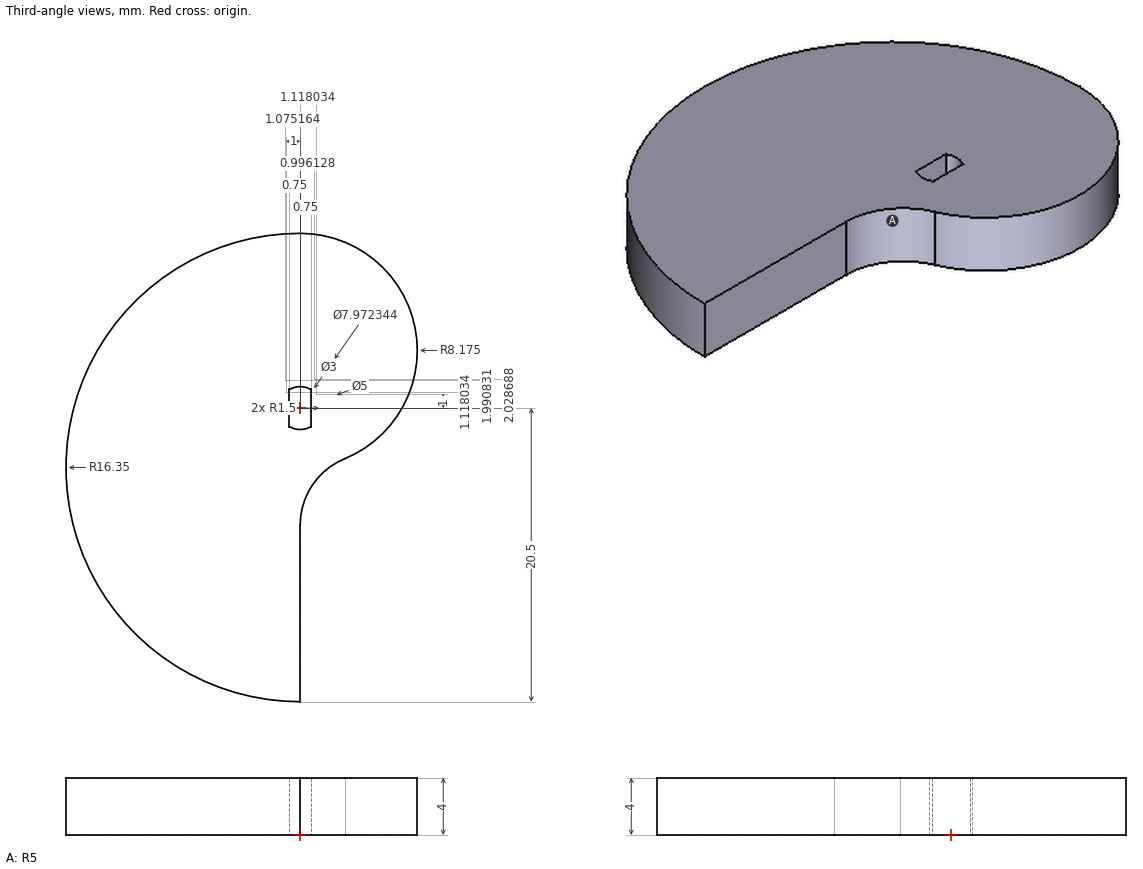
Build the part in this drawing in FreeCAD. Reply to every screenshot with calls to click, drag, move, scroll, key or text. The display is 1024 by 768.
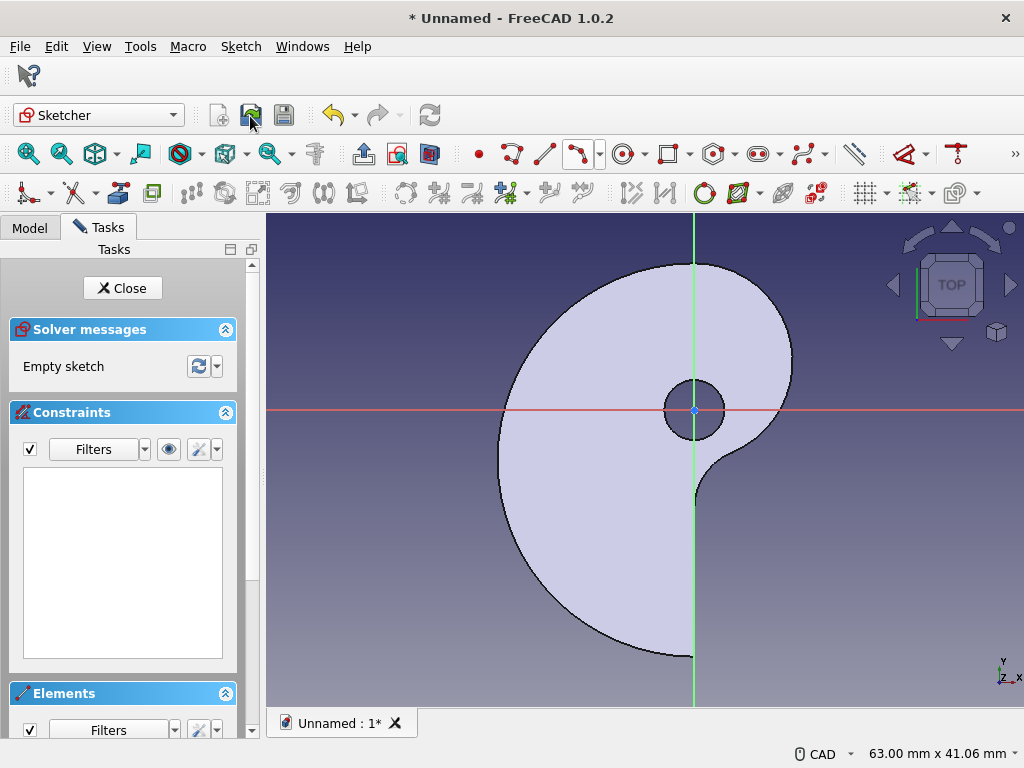
scroll(745, 389, up, 6)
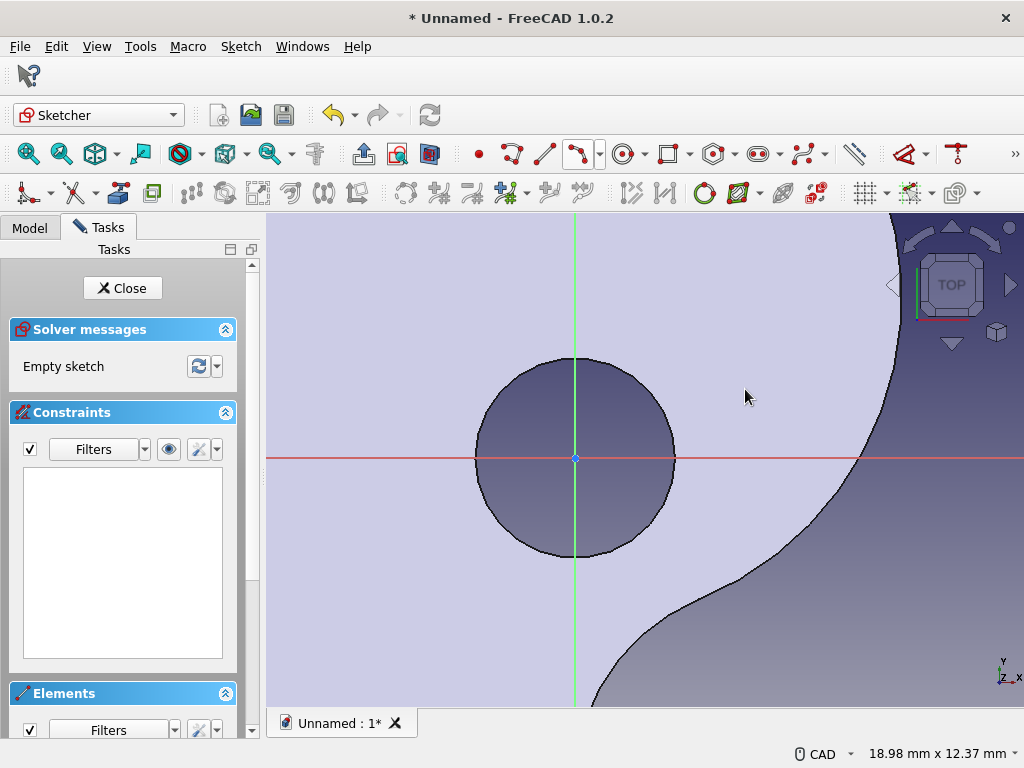
click(622, 154)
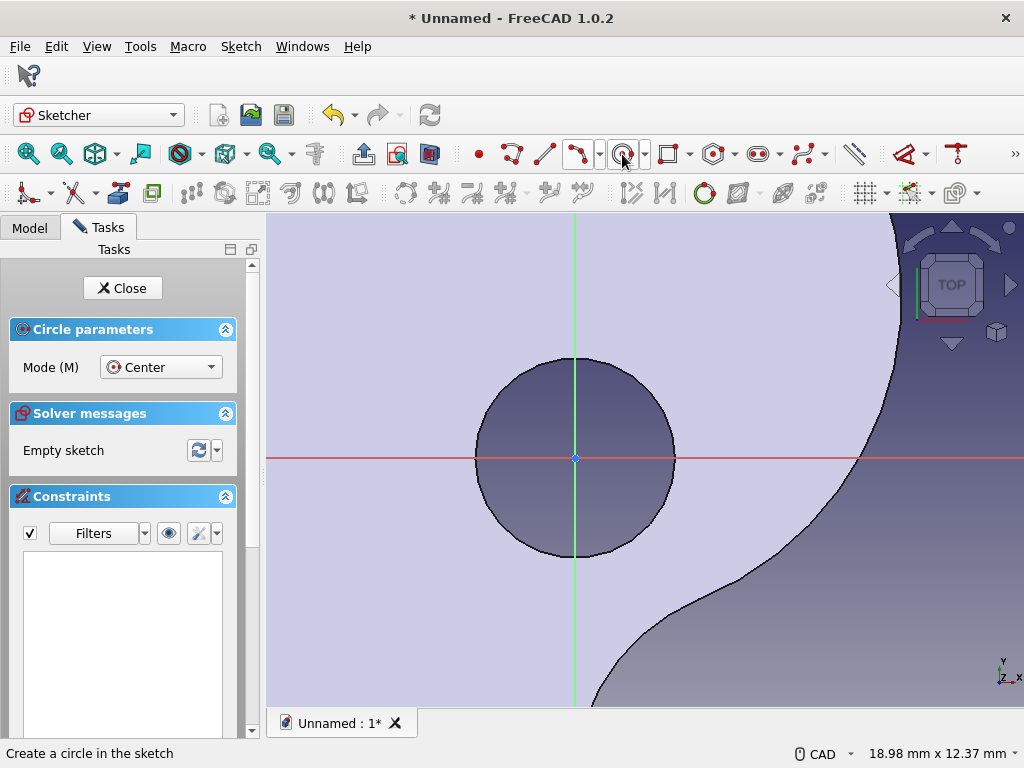
click(575, 458)
move(688, 346)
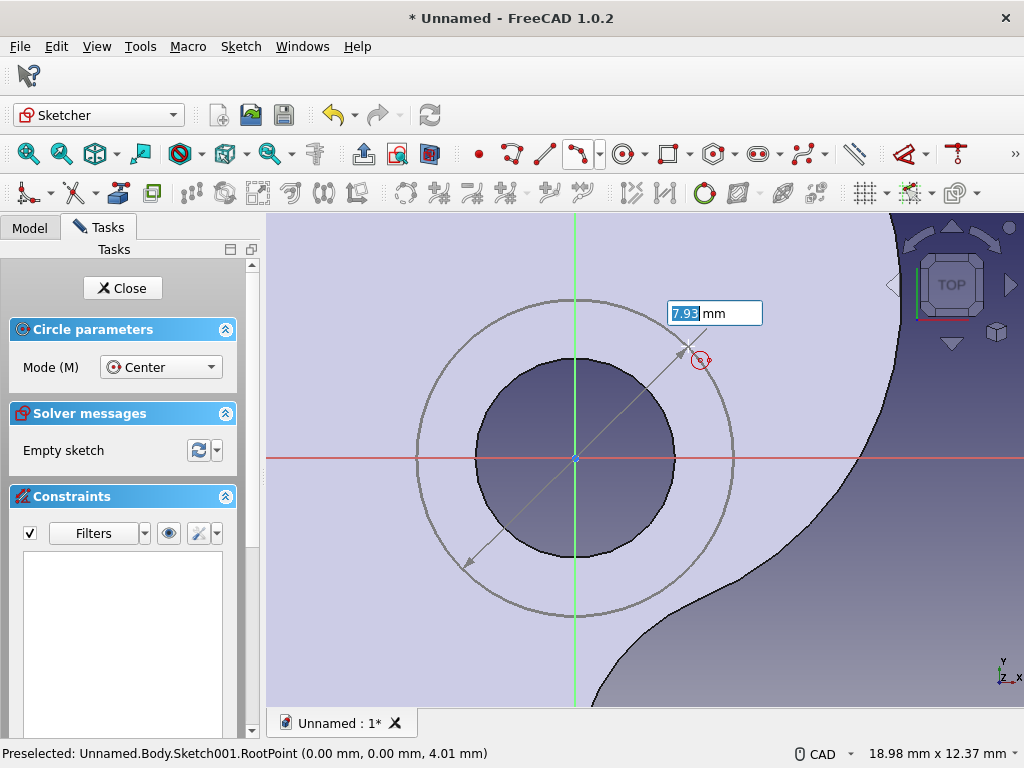
text(7.972344)
key(Return)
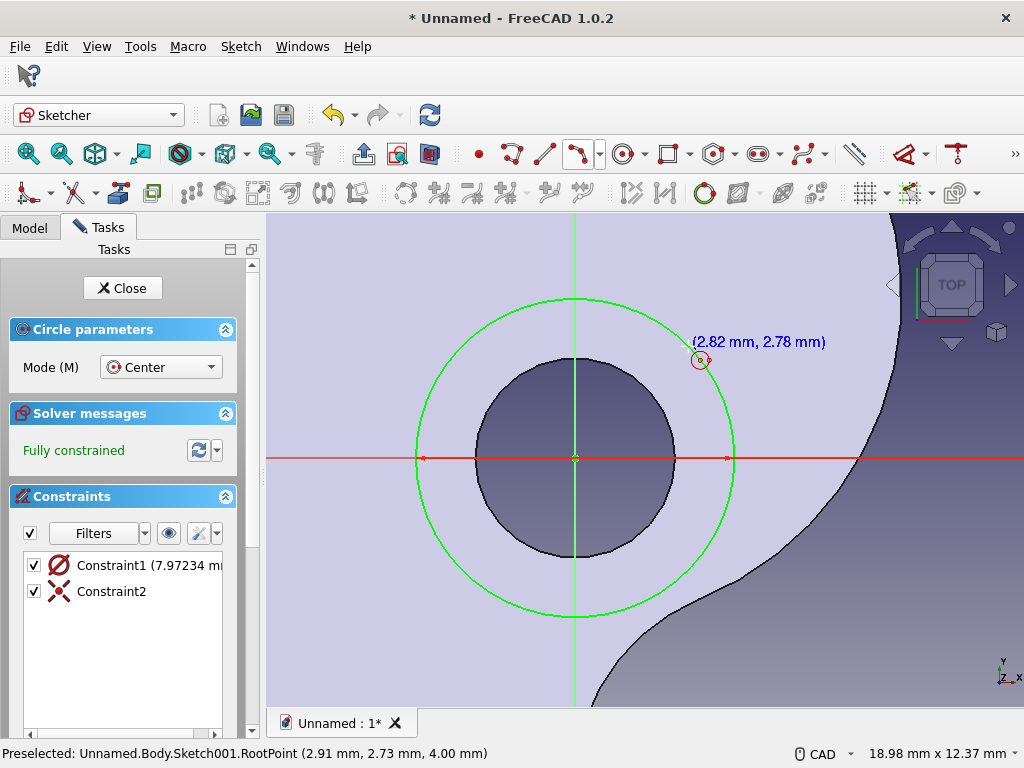
click(575, 458)
move(618, 416)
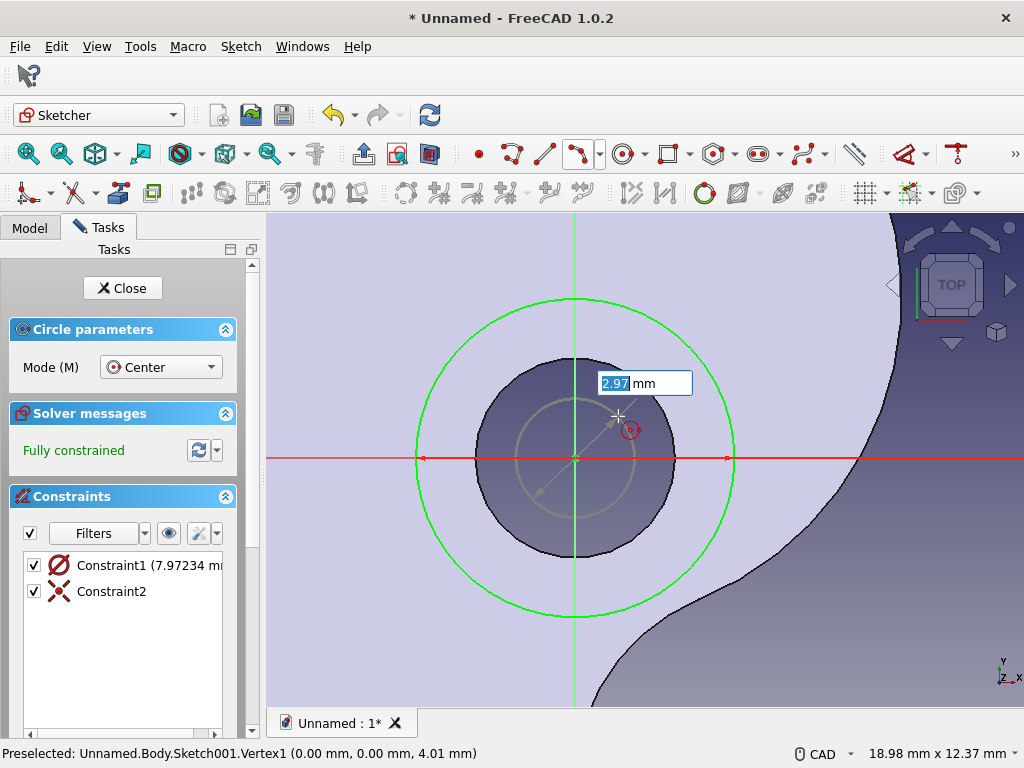
text(3)
key(Return)
key(Escape)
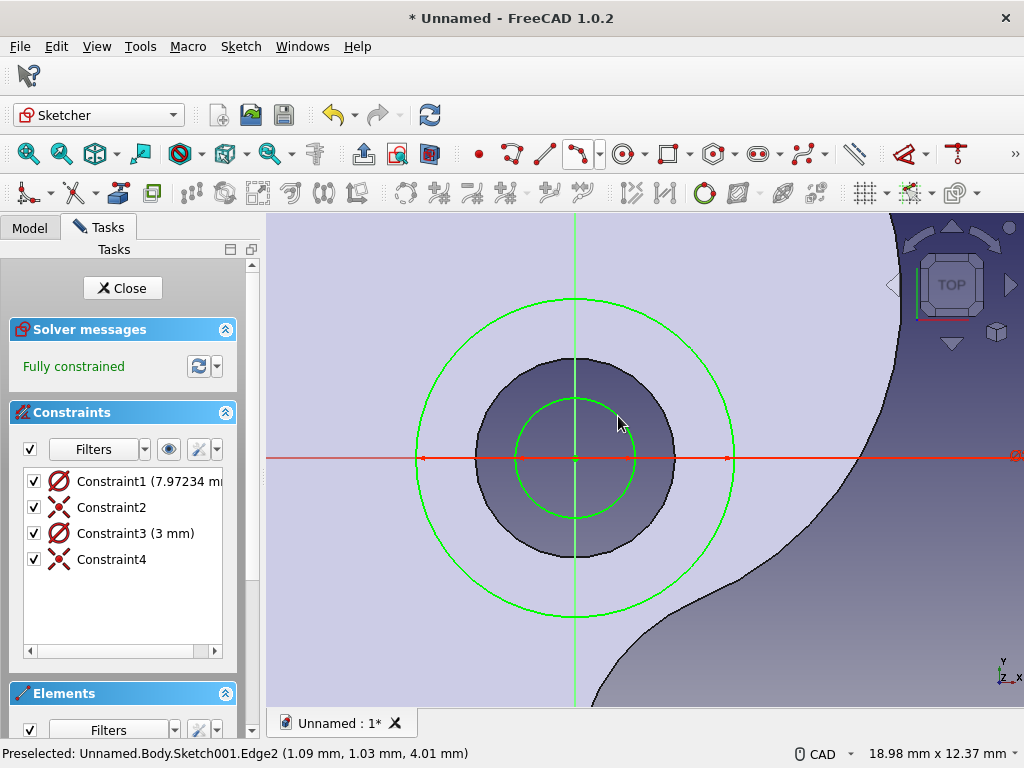
click(123, 288)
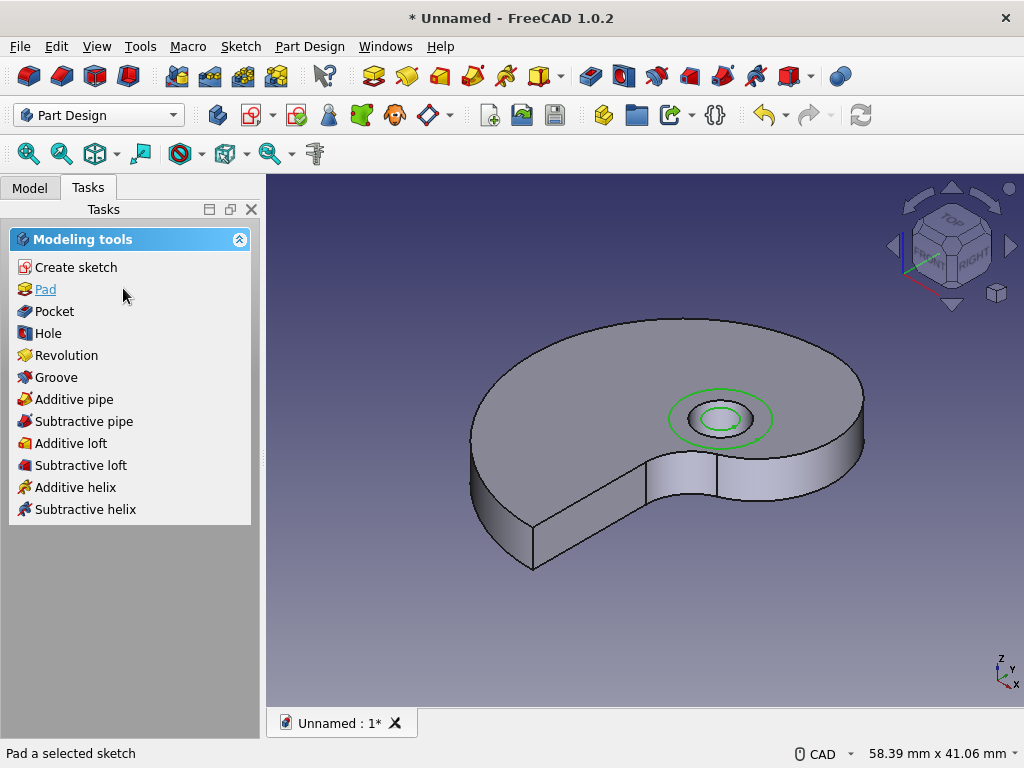
click(374, 76)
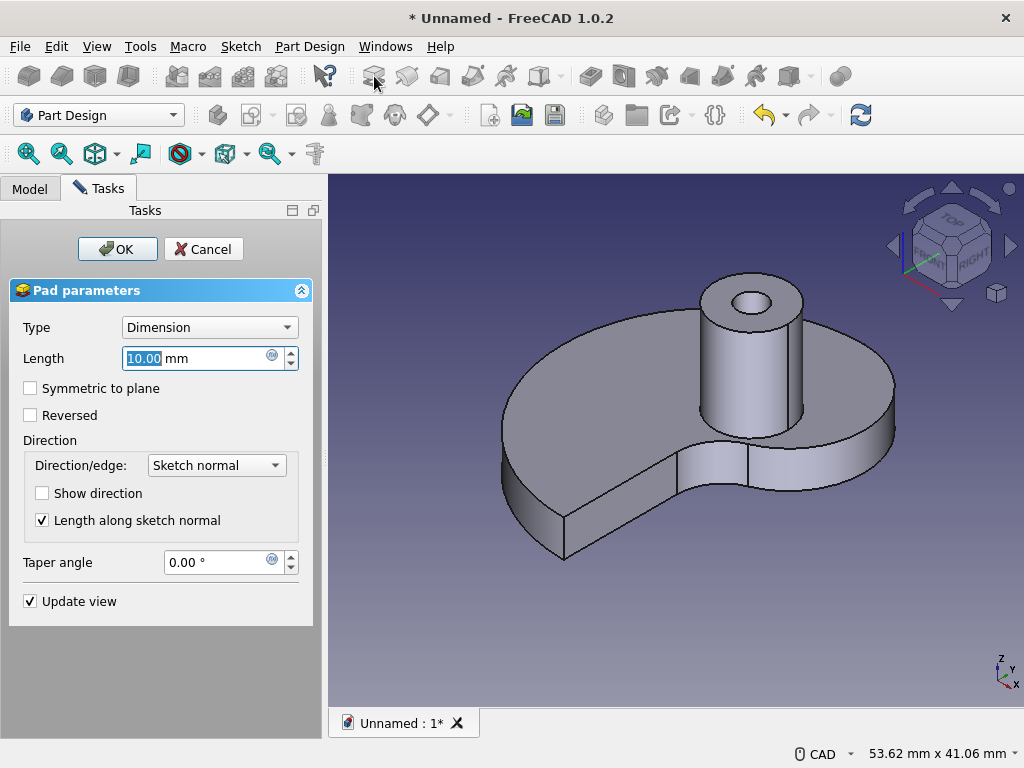
text(4)
key(Tab)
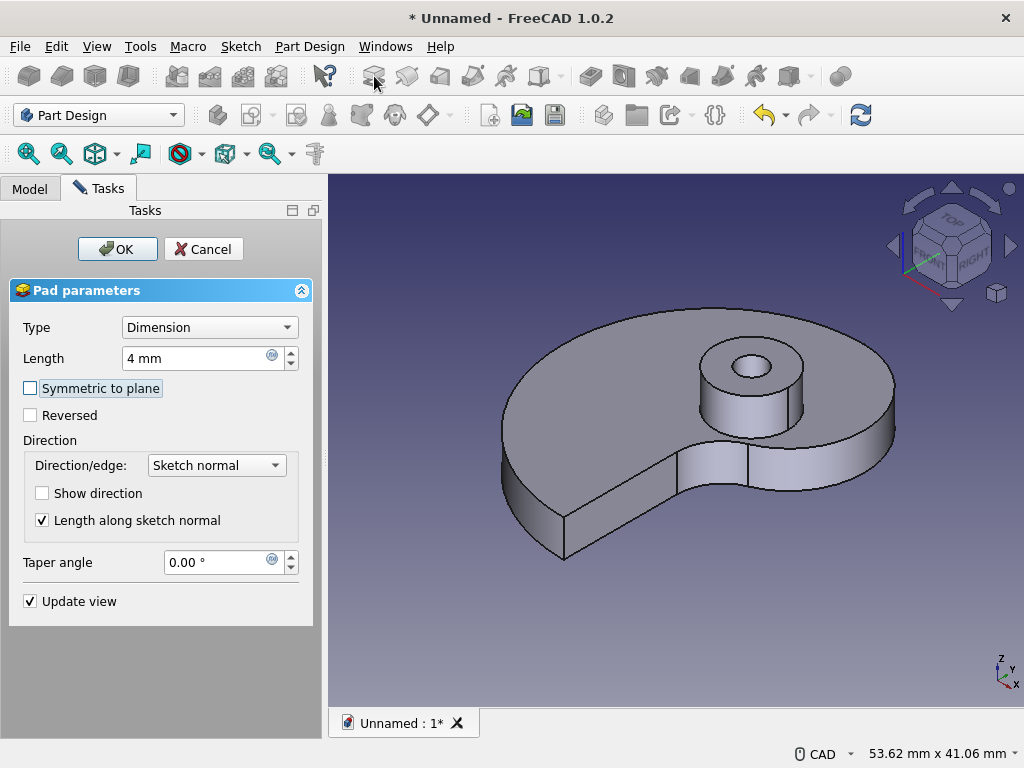
click(31, 415)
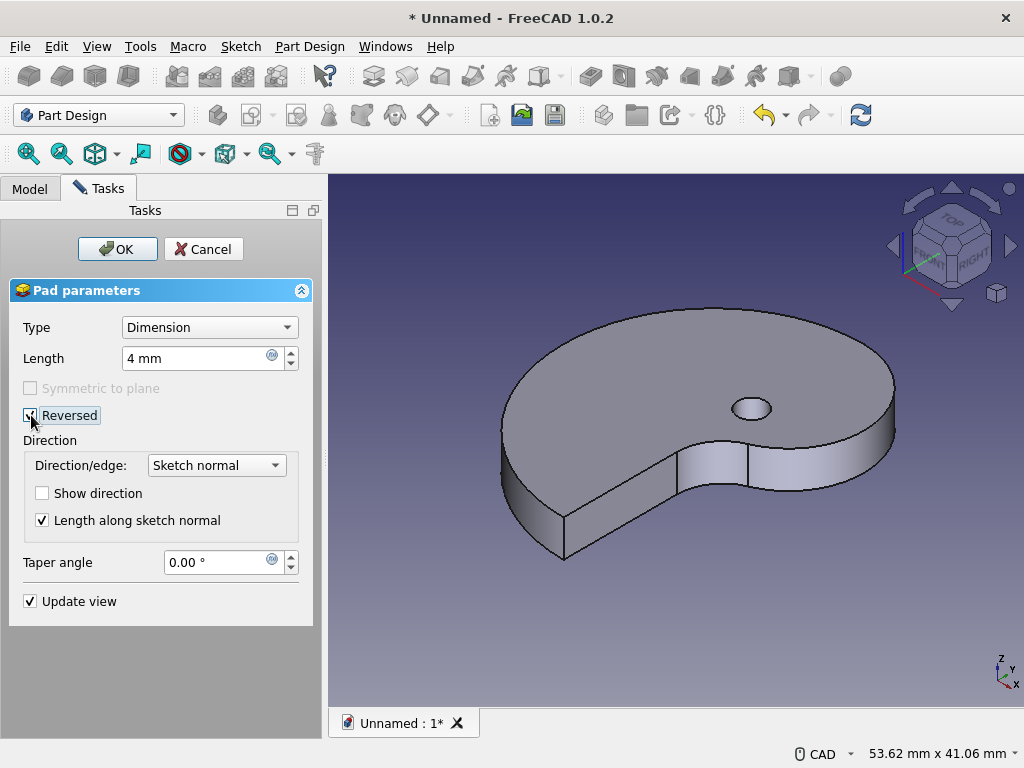
click(118, 249)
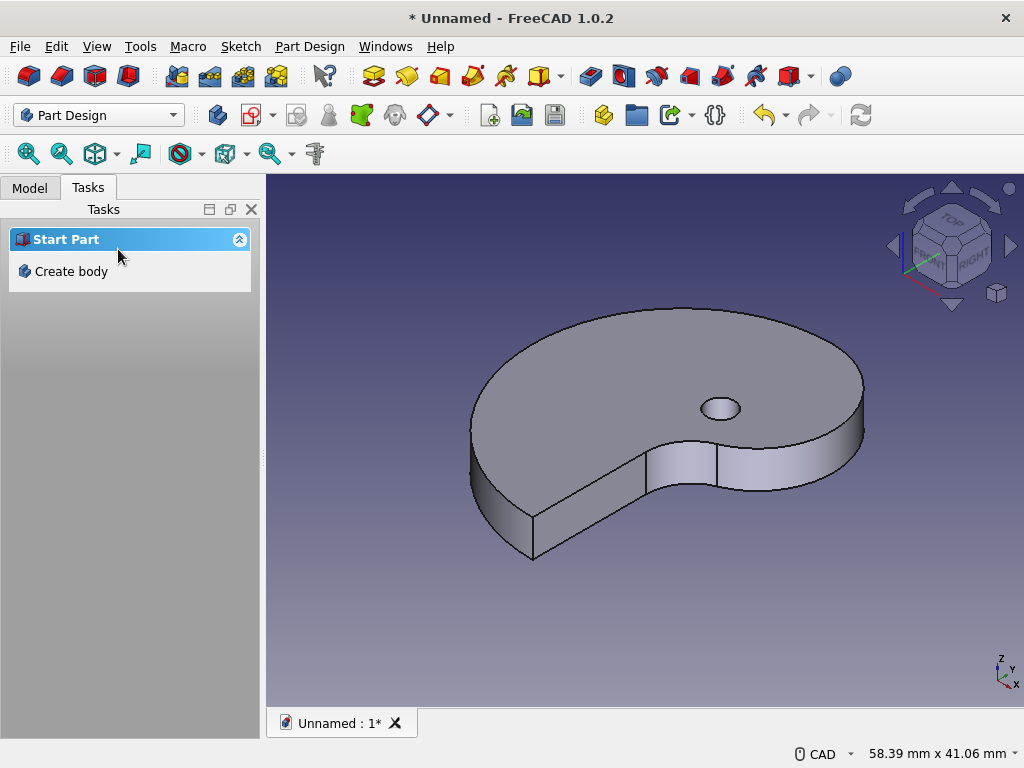
click(570, 414)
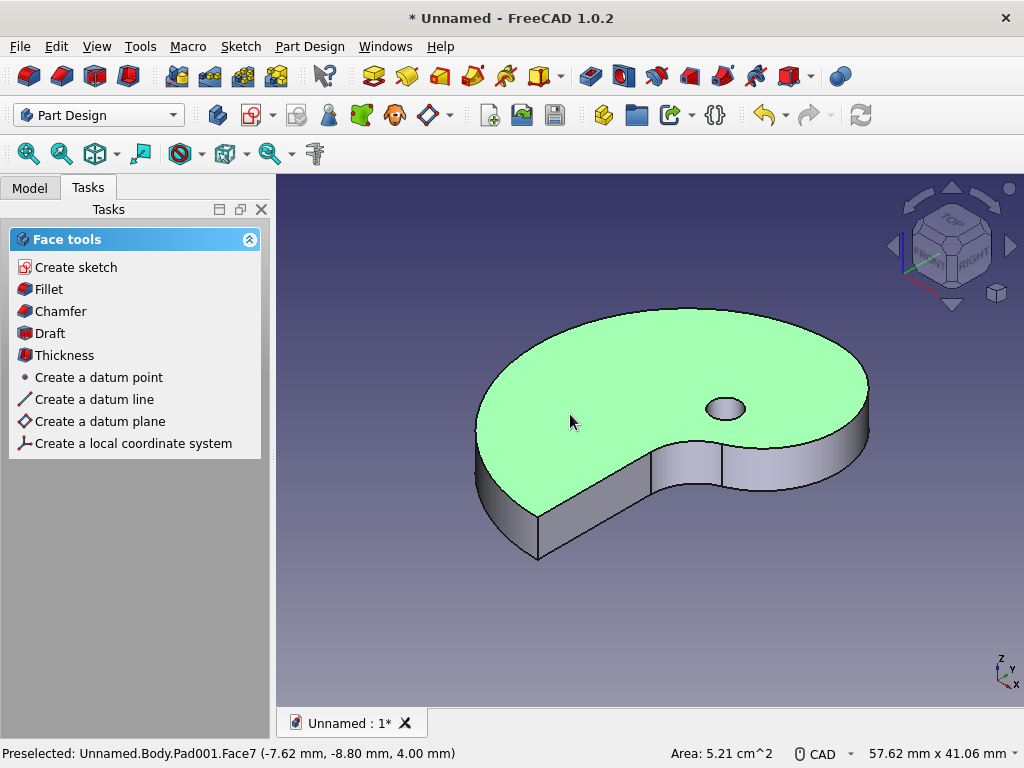
click(250, 116)